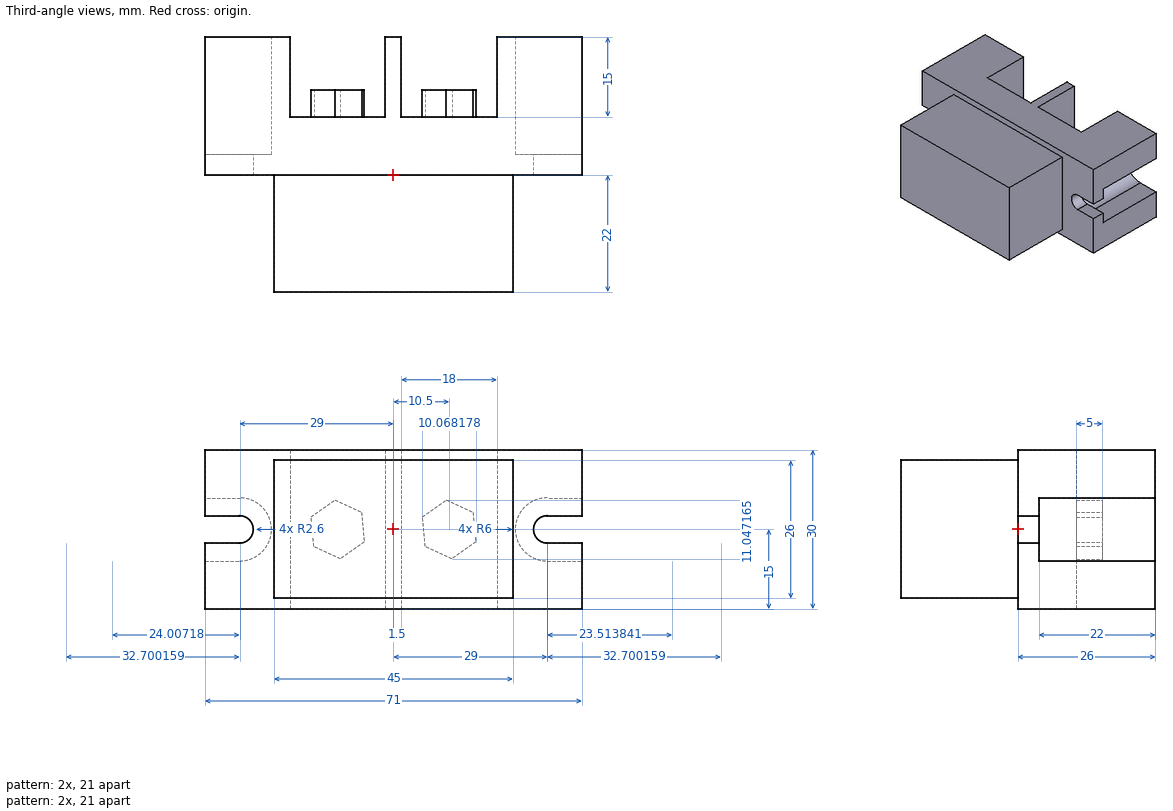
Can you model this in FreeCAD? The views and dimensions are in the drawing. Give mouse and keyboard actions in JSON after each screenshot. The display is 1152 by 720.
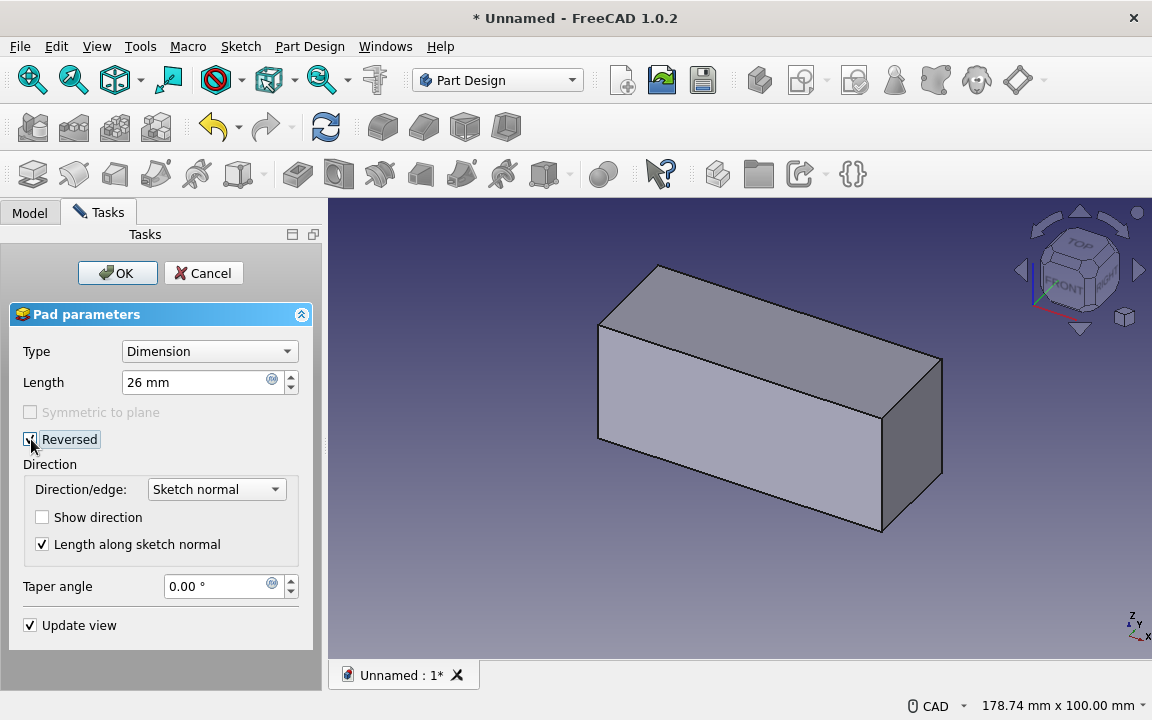
{"action": "left_click", "coordinate": [118, 273]}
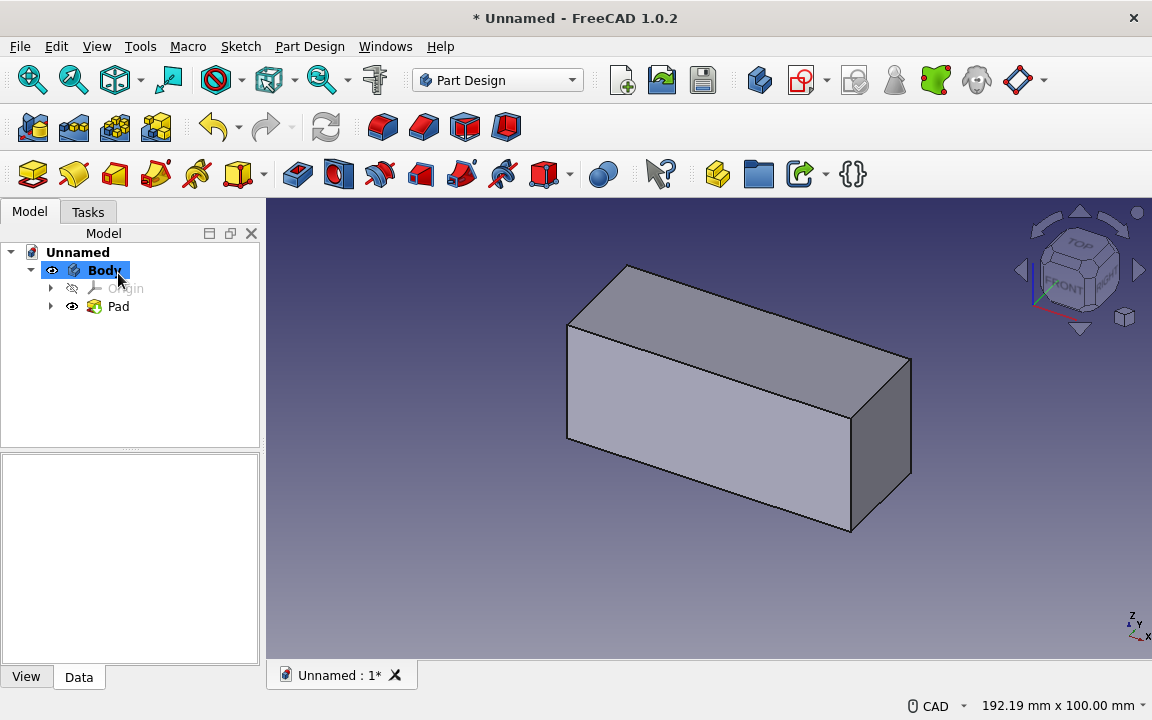
{"action": "left_click", "coordinate": [800, 80]}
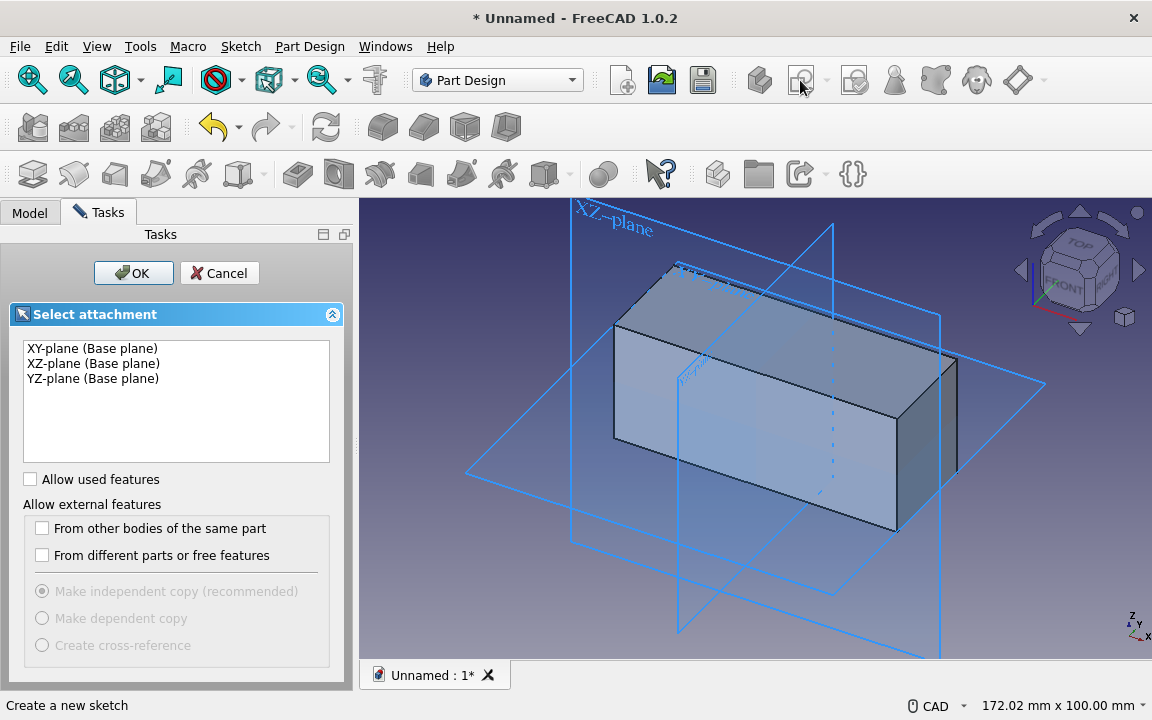
{"action": "left_click", "coordinate": [84, 364]}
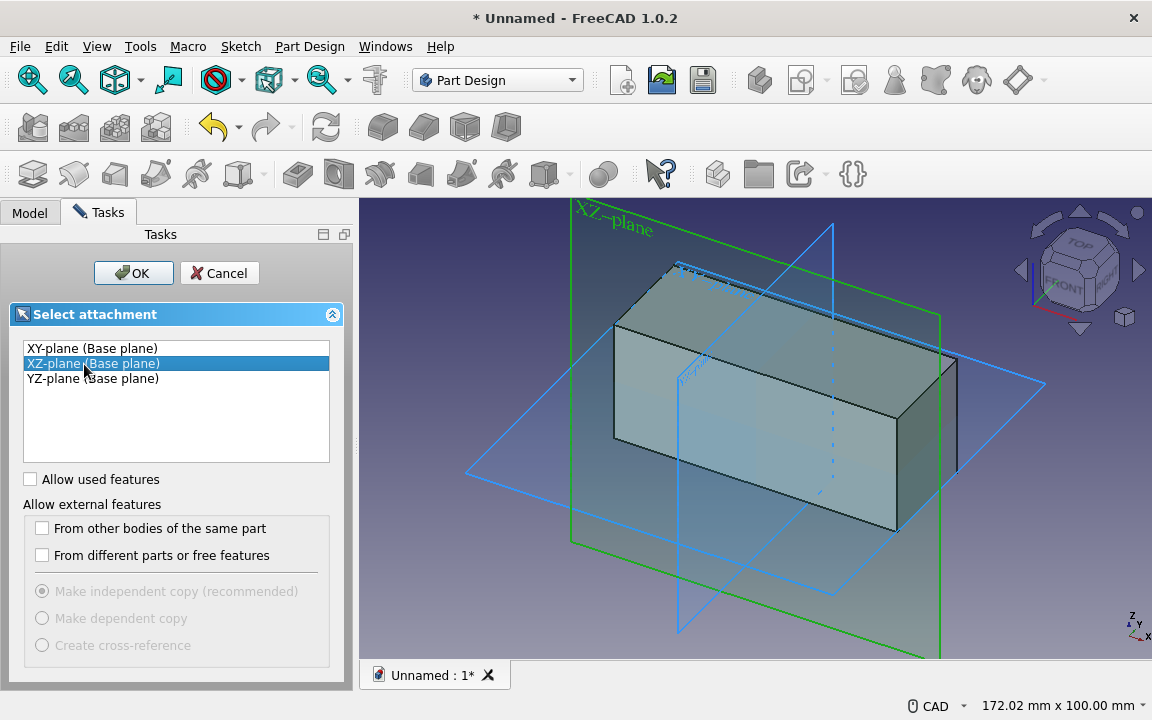
{"action": "left_click", "coordinate": [134, 273]}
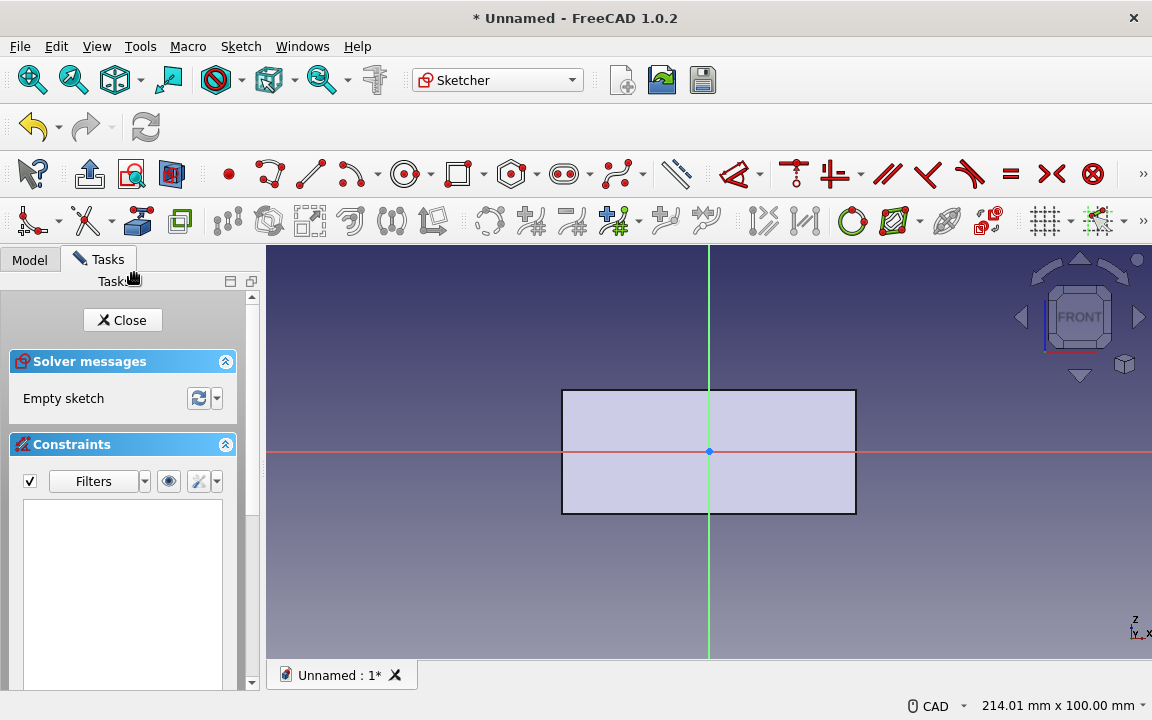
{"action": "scroll", "coordinate": [765, 452], "scroll_direction": "up", "scroll_amount": 4}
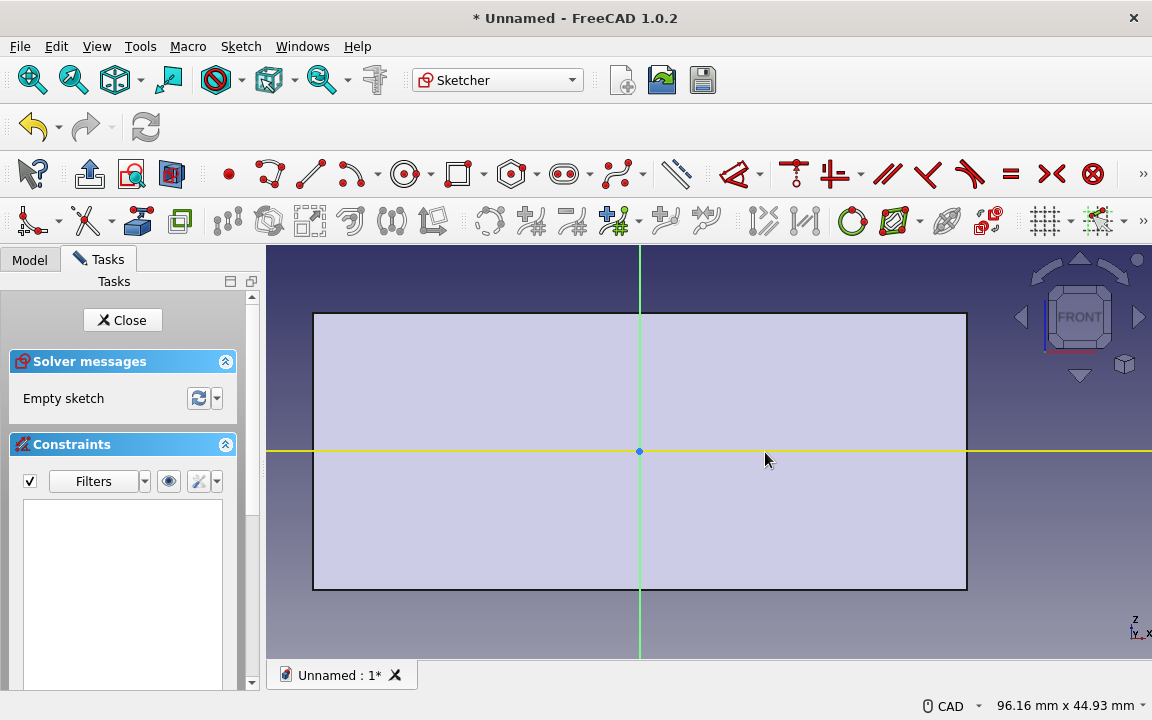
{"action": "left_click", "coordinate": [484, 174]}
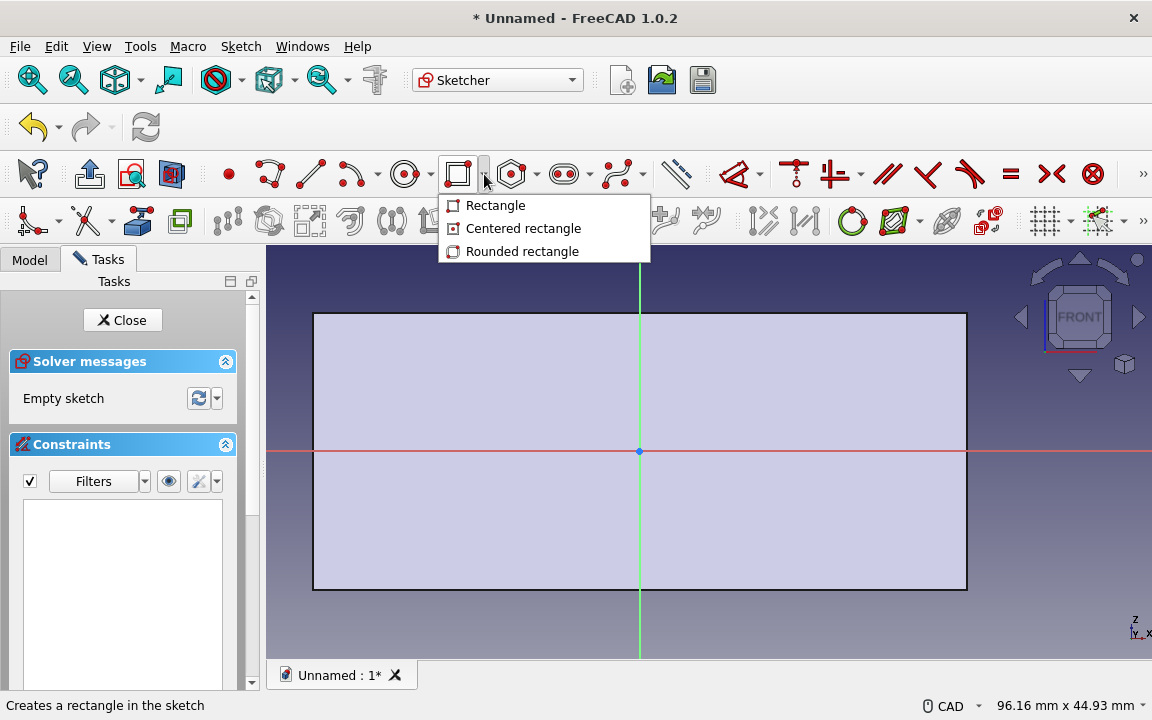
{"action": "left_click", "coordinate": [544, 228]}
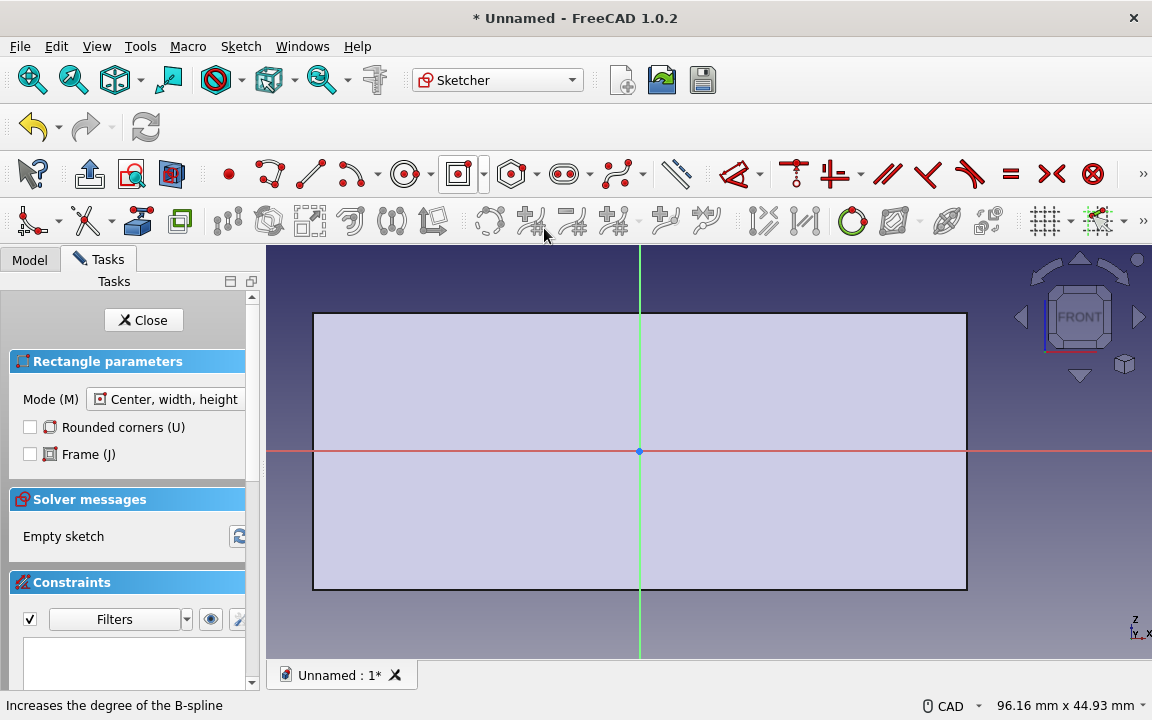
{"action": "left_click", "coordinate": [640, 451]}
{"action": "mouse_move", "coordinate": [847, 332]}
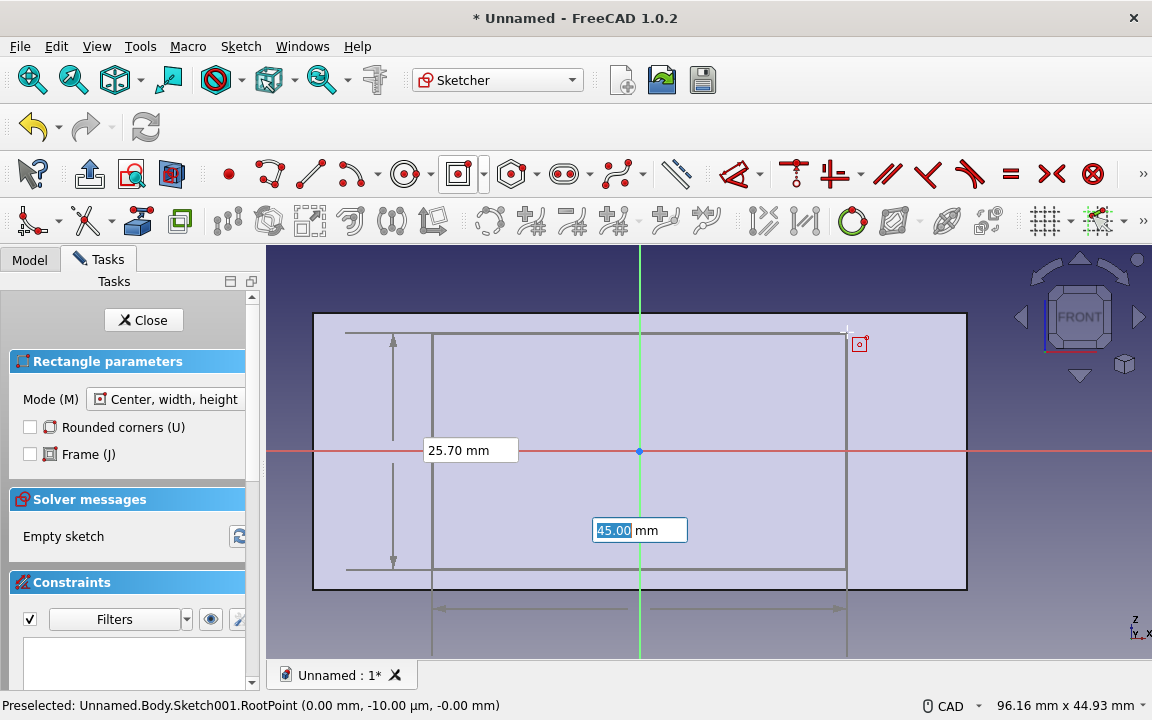
{"action": "type", "text": "45"}
{"action": "key", "text": "Tab"}
{"action": "type", "text": "26"}
{"action": "key", "text": "Return"}
{"action": "key", "text": "Escape"}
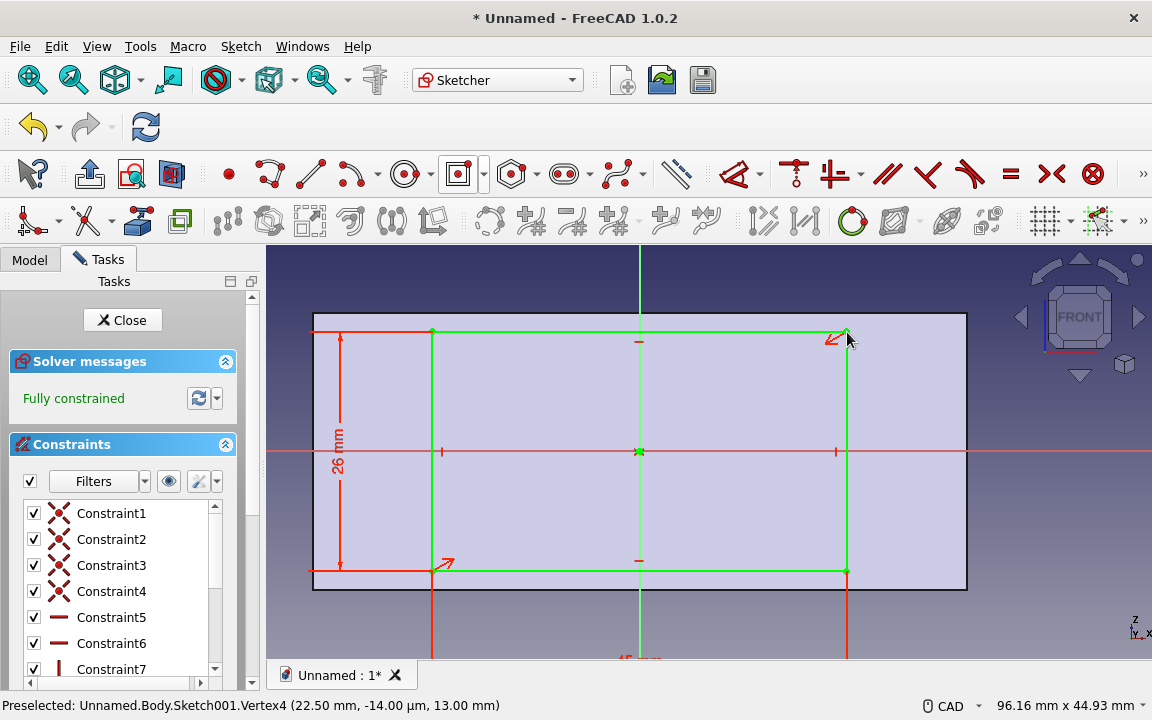
{"action": "left_click", "coordinate": [123, 320]}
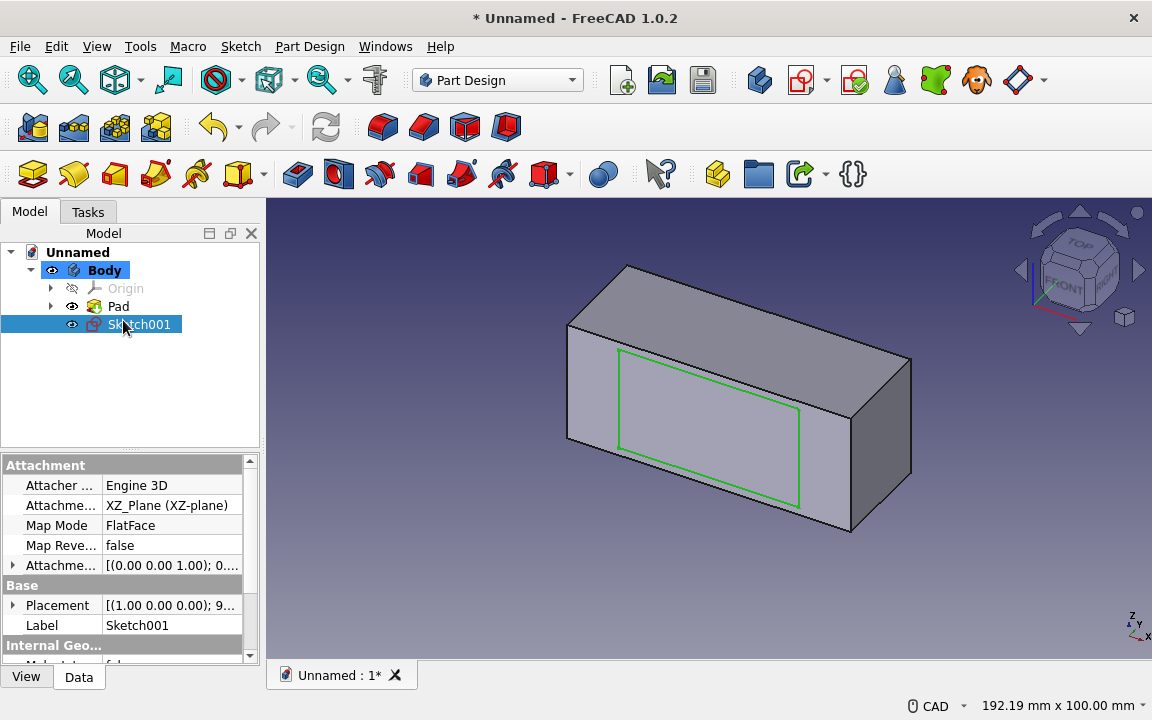
{"action": "left_click", "coordinate": [33, 174]}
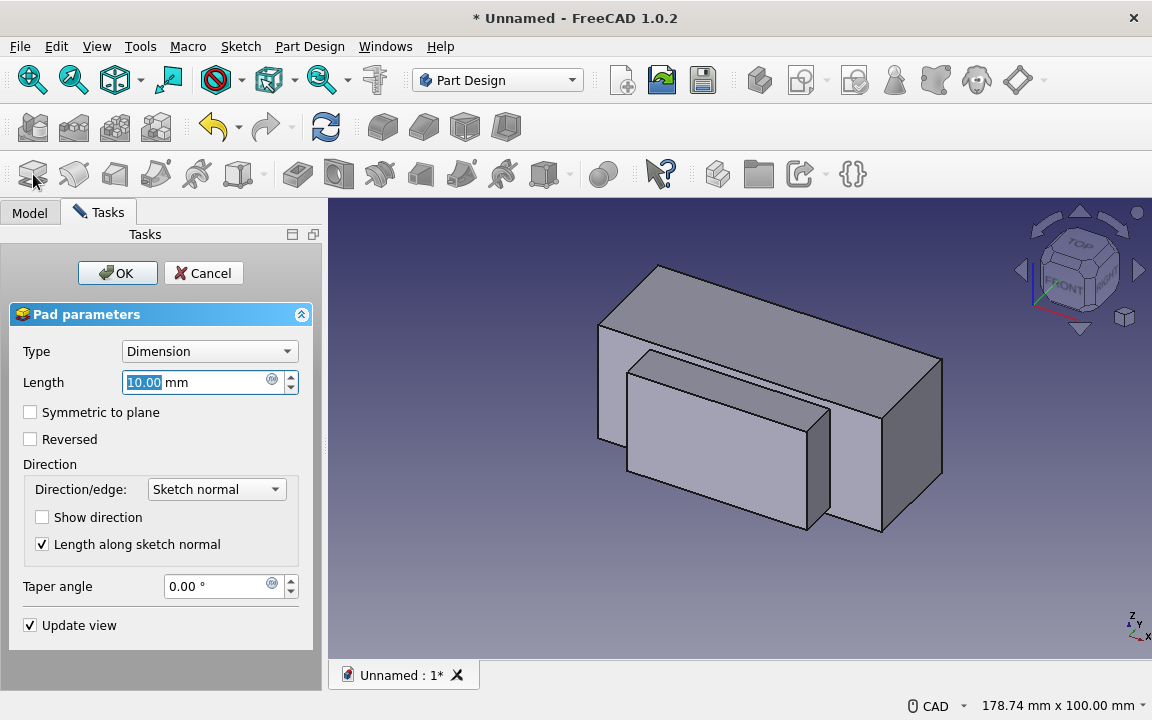
{"action": "type", "text": "22"}
{"action": "key", "text": "Tab"}